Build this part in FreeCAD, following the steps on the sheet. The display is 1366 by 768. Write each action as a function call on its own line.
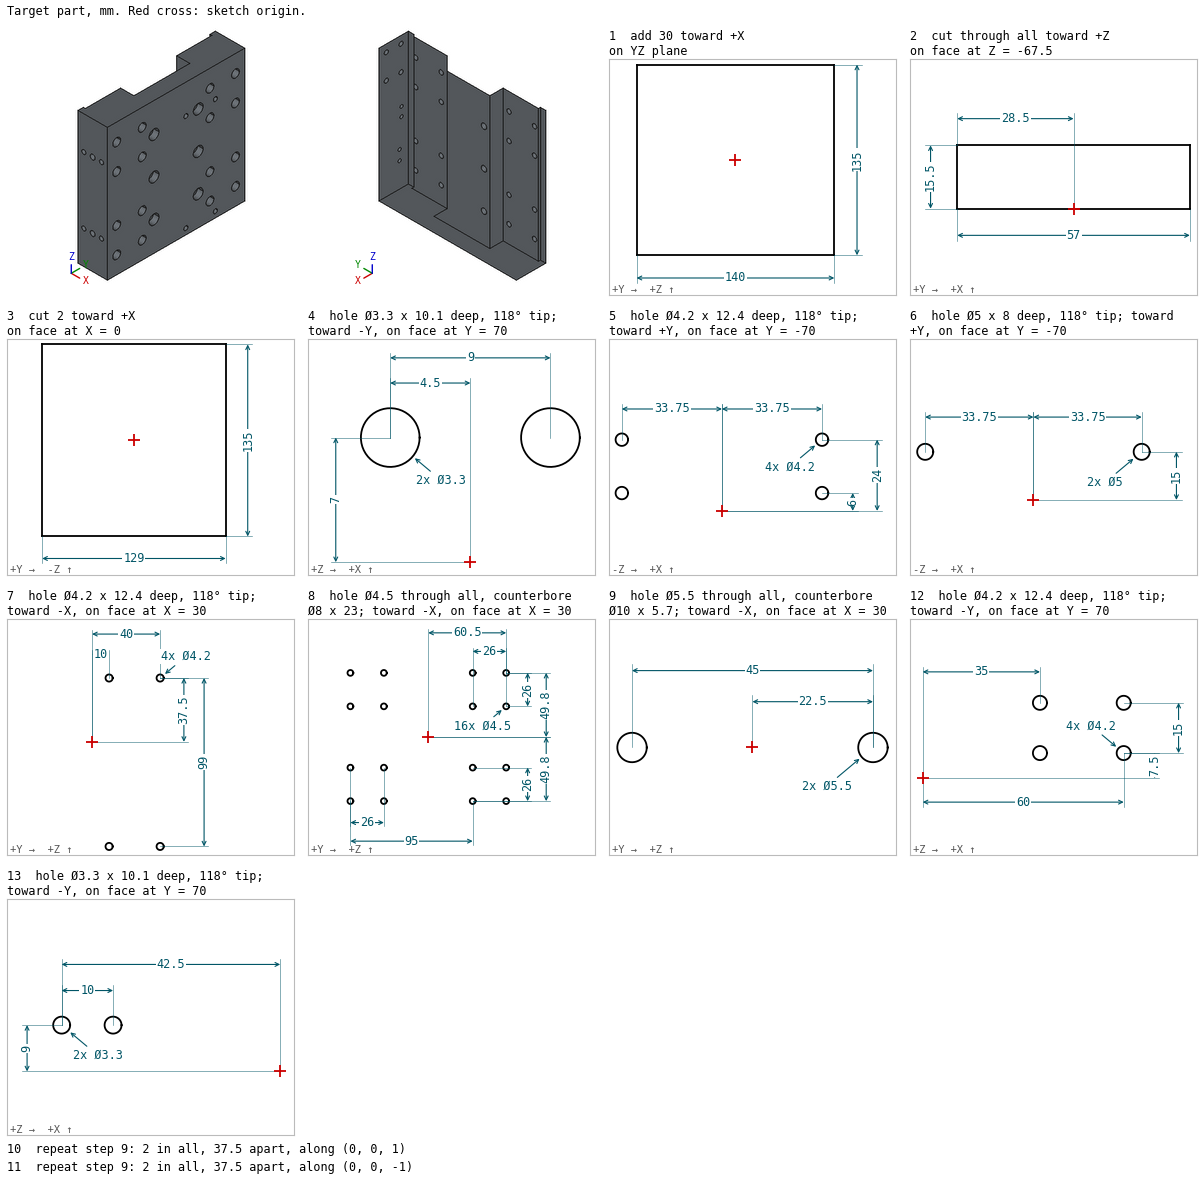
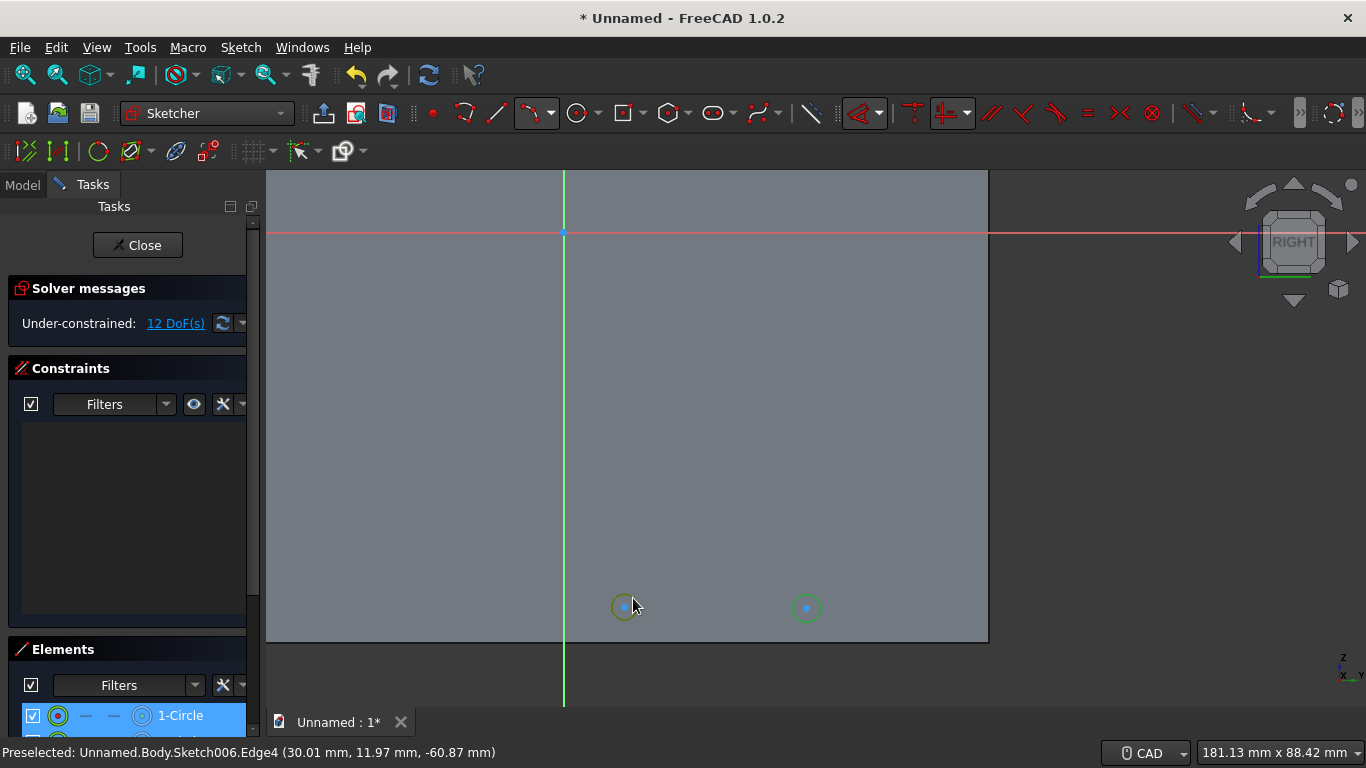
click(1088, 114)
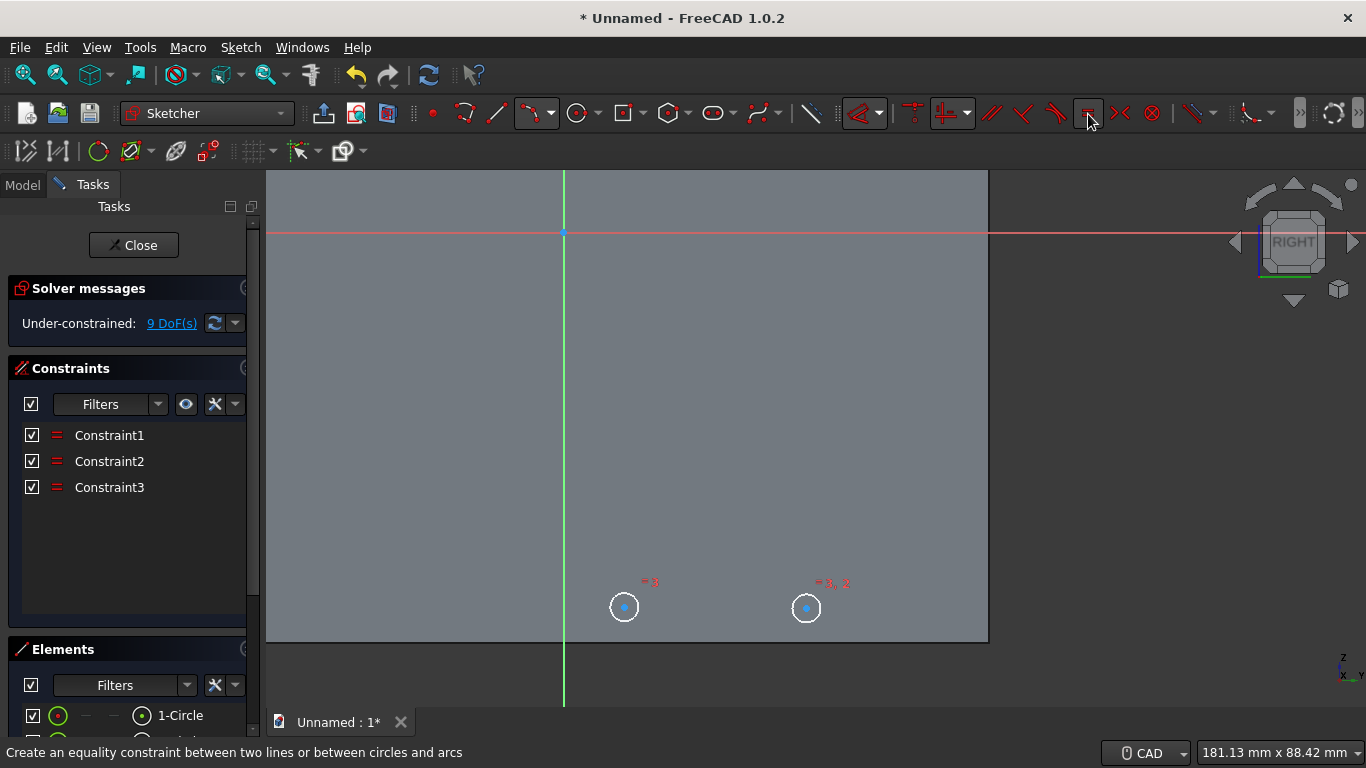
scroll(816, 600, down, 3)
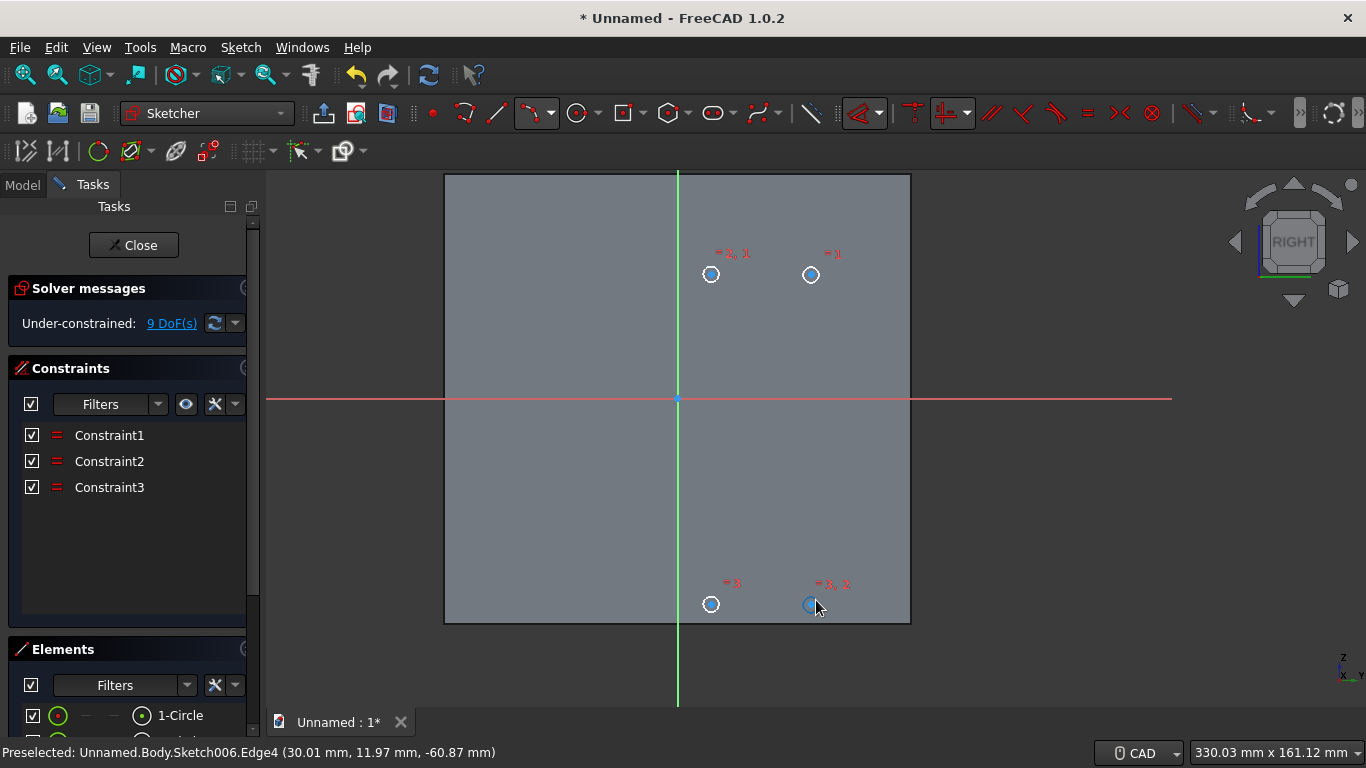
click(811, 275)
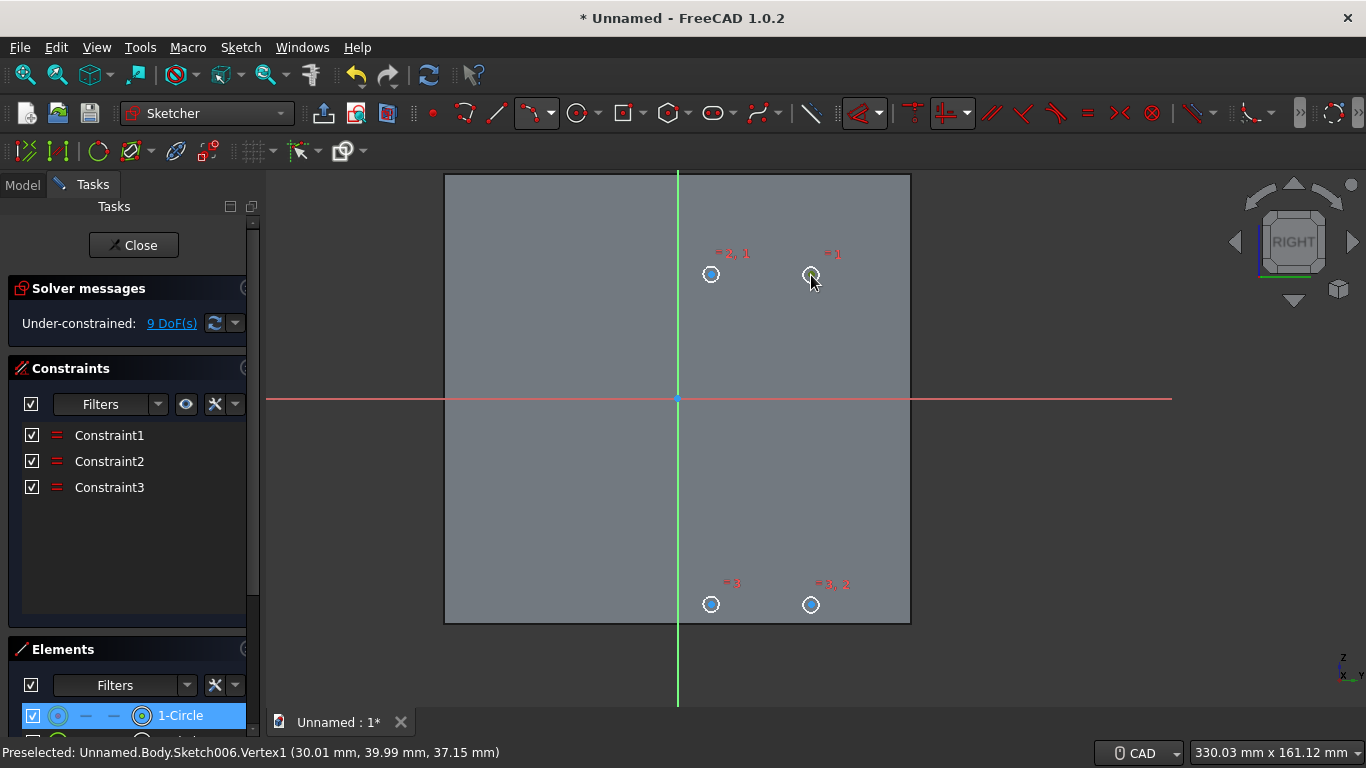
click(711, 274)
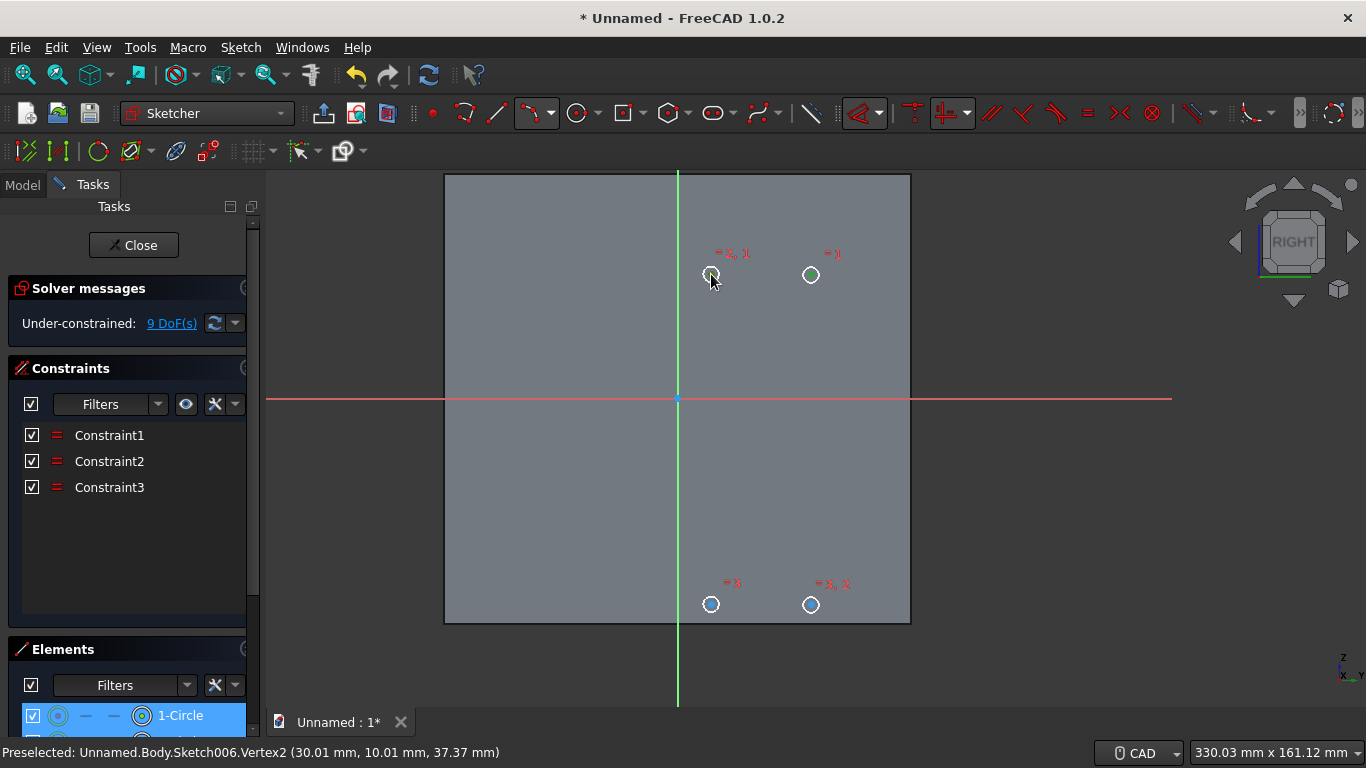
key(h)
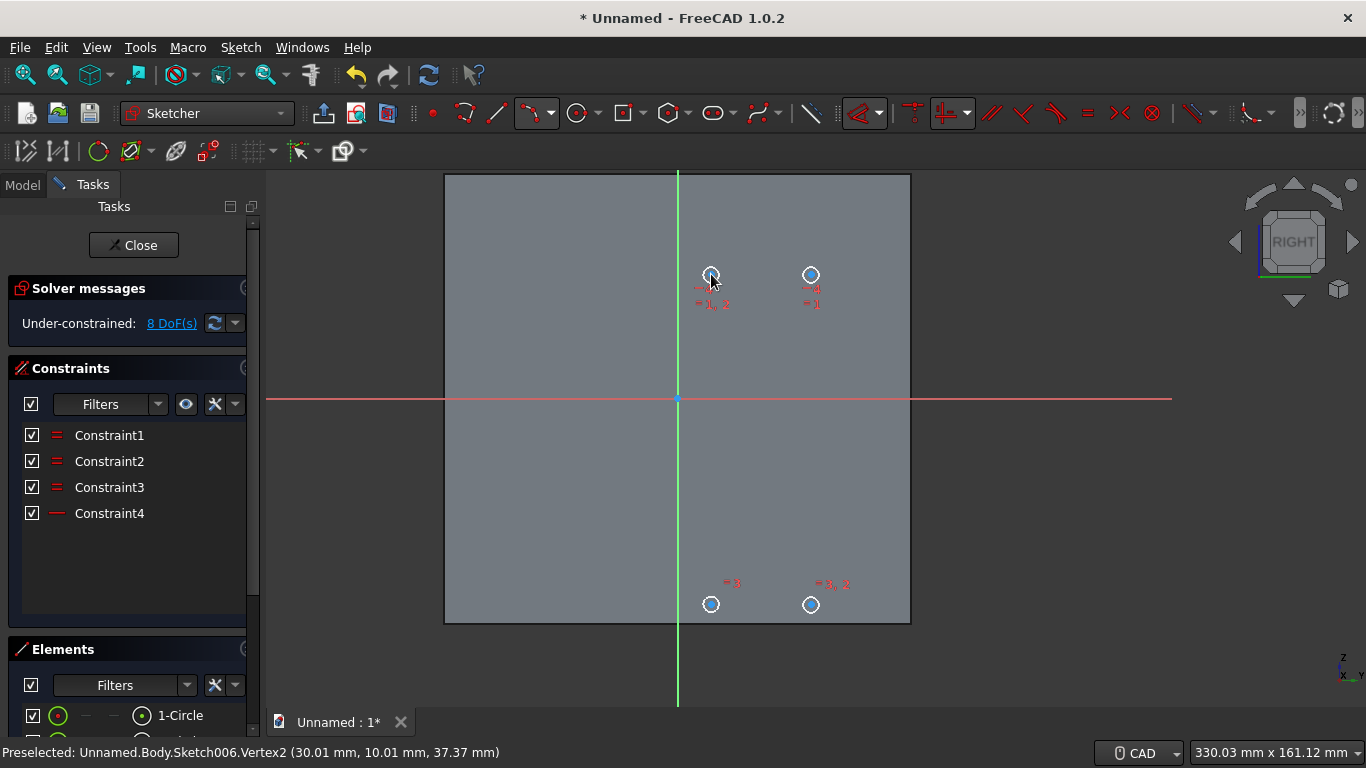
click(811, 275)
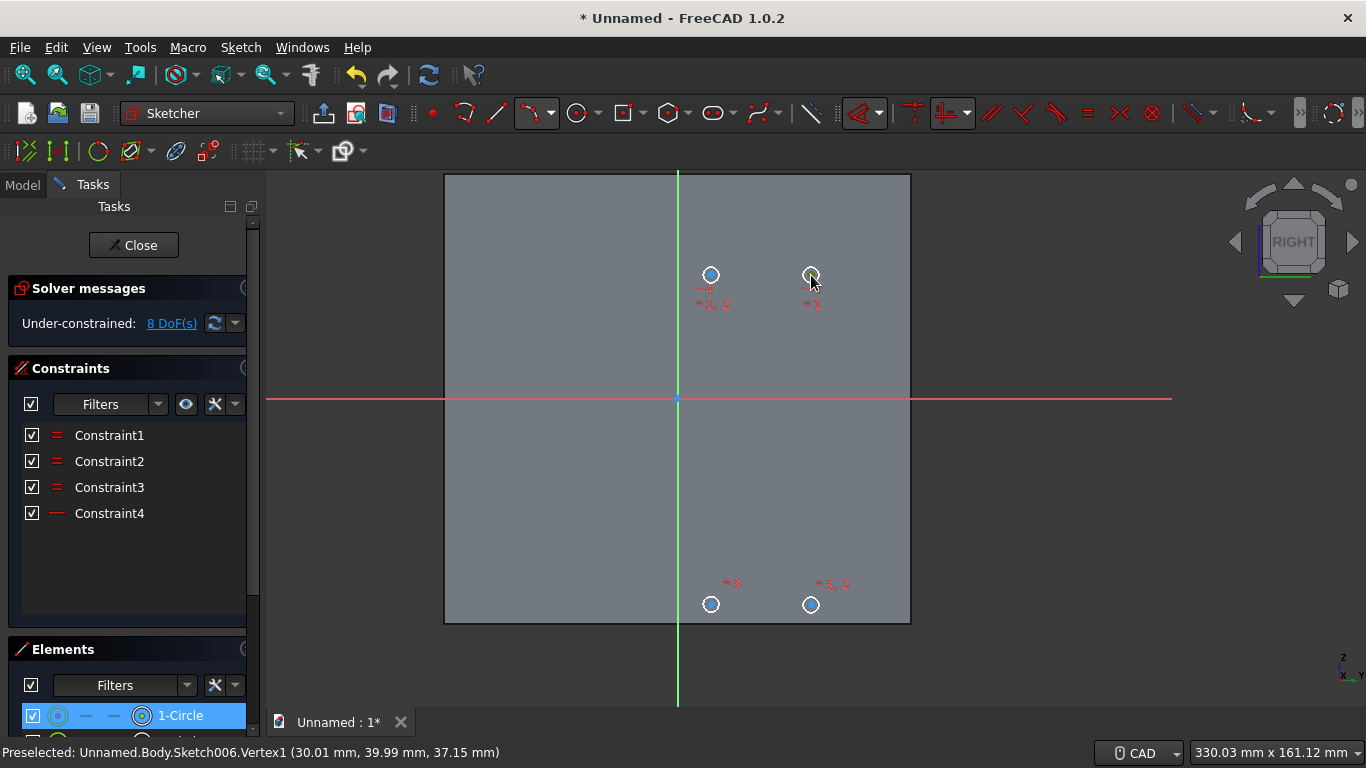
click(811, 605)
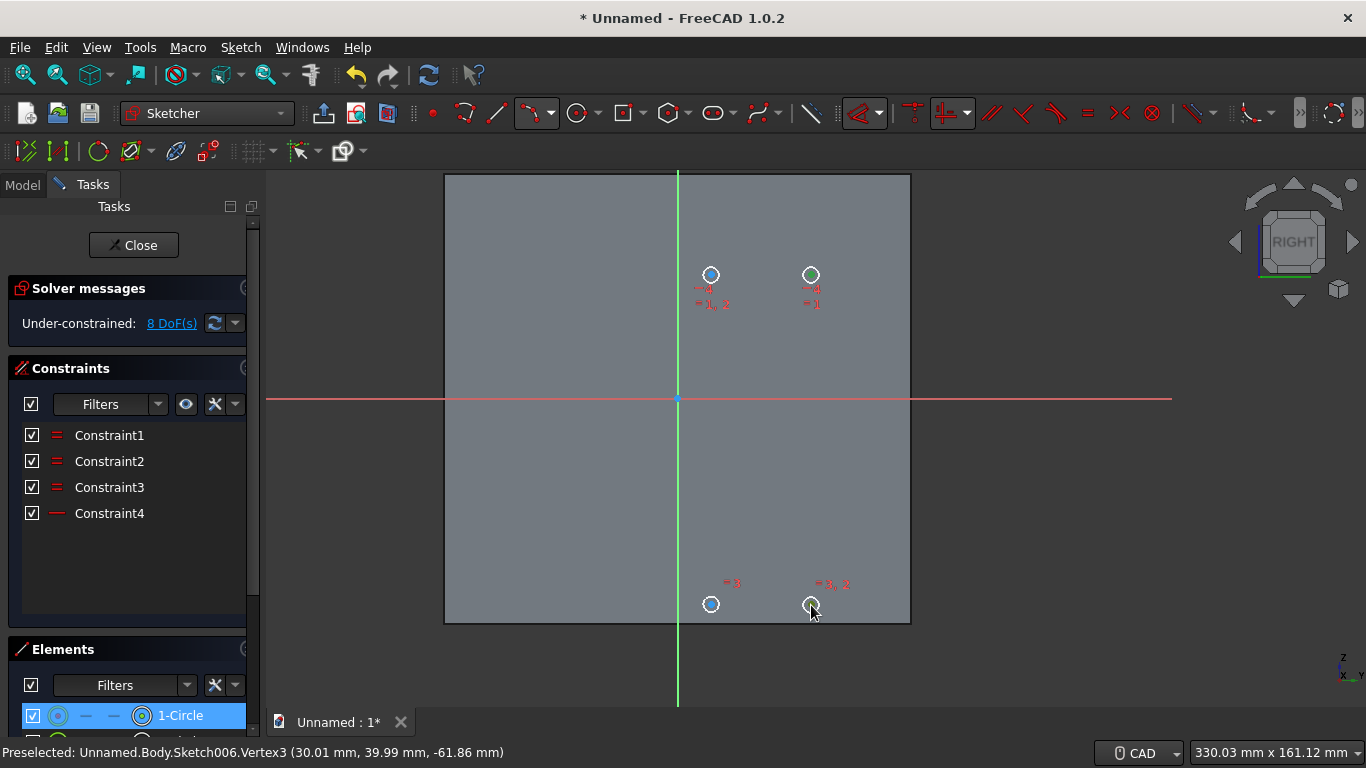
key(v)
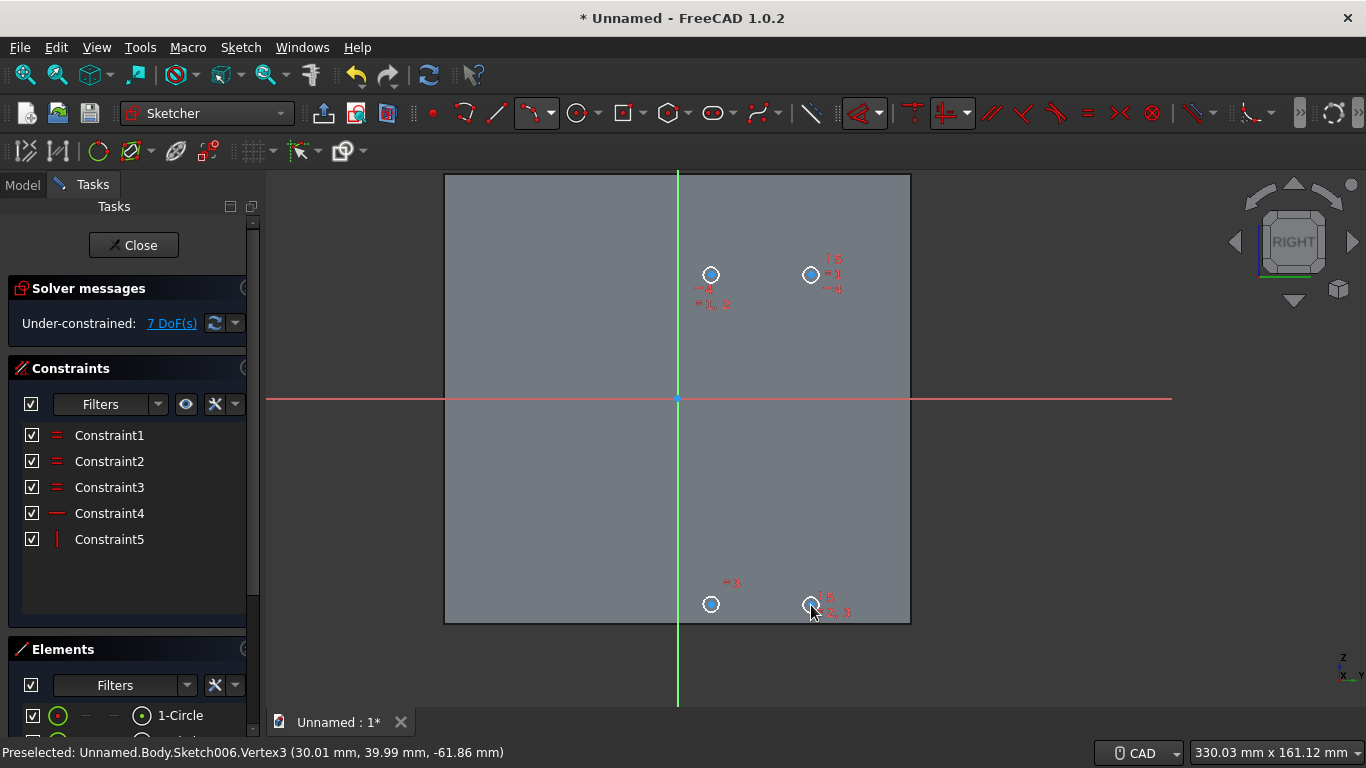
click(711, 275)